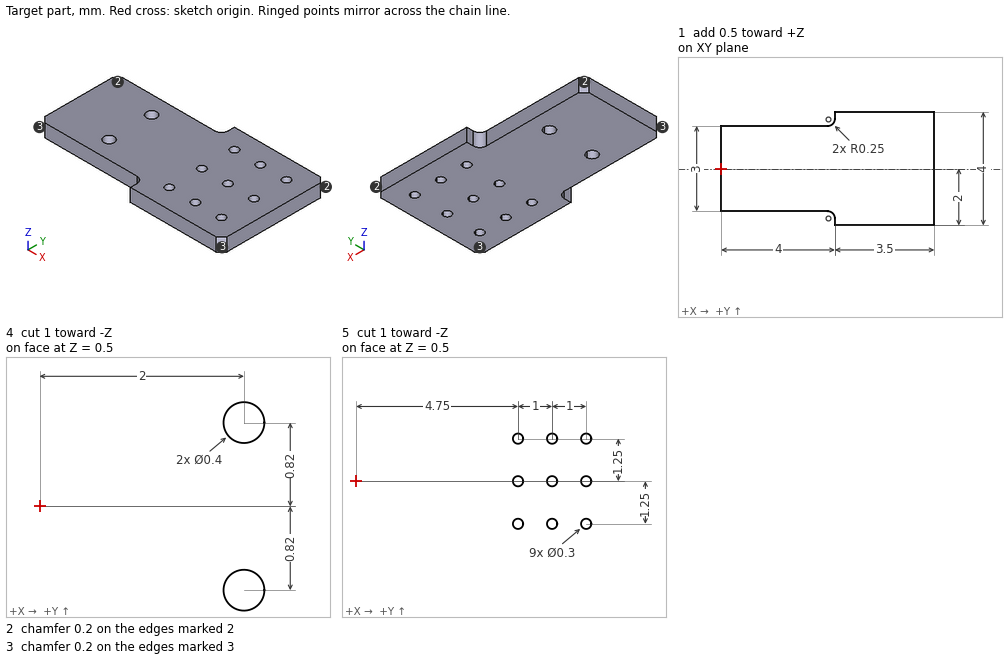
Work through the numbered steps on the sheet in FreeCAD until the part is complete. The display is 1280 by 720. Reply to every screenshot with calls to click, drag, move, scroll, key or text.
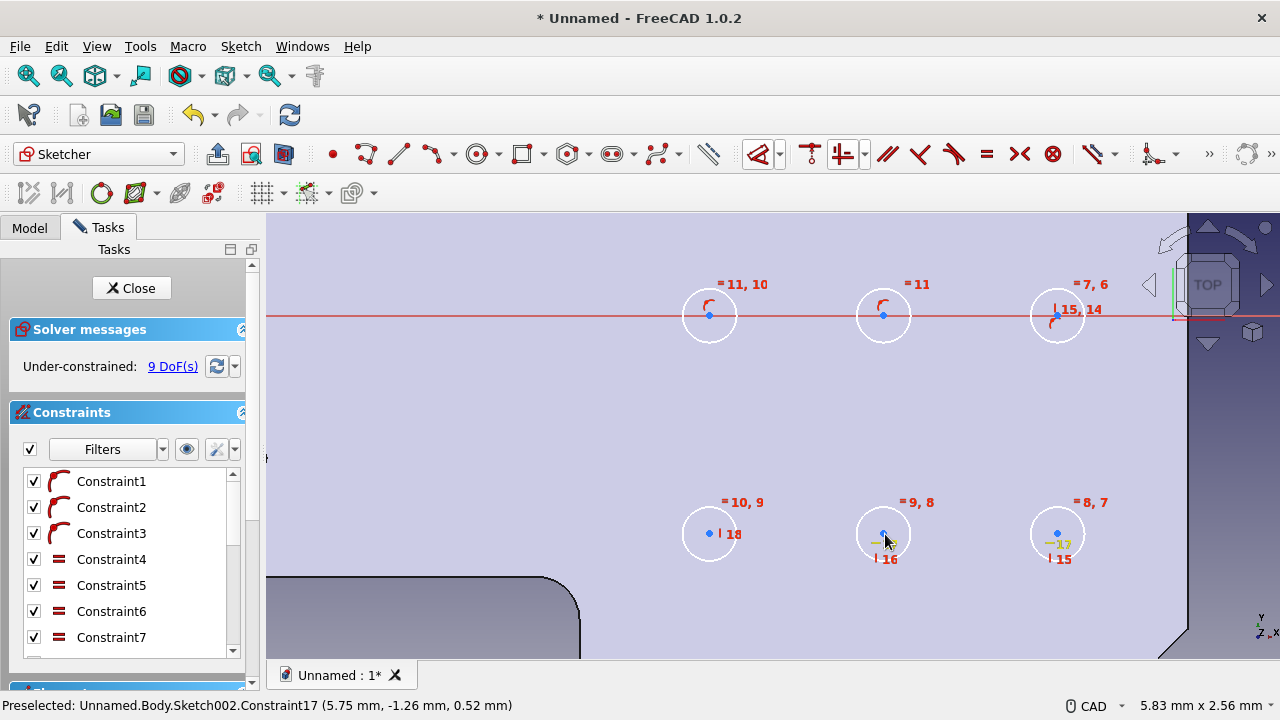
click(884, 534)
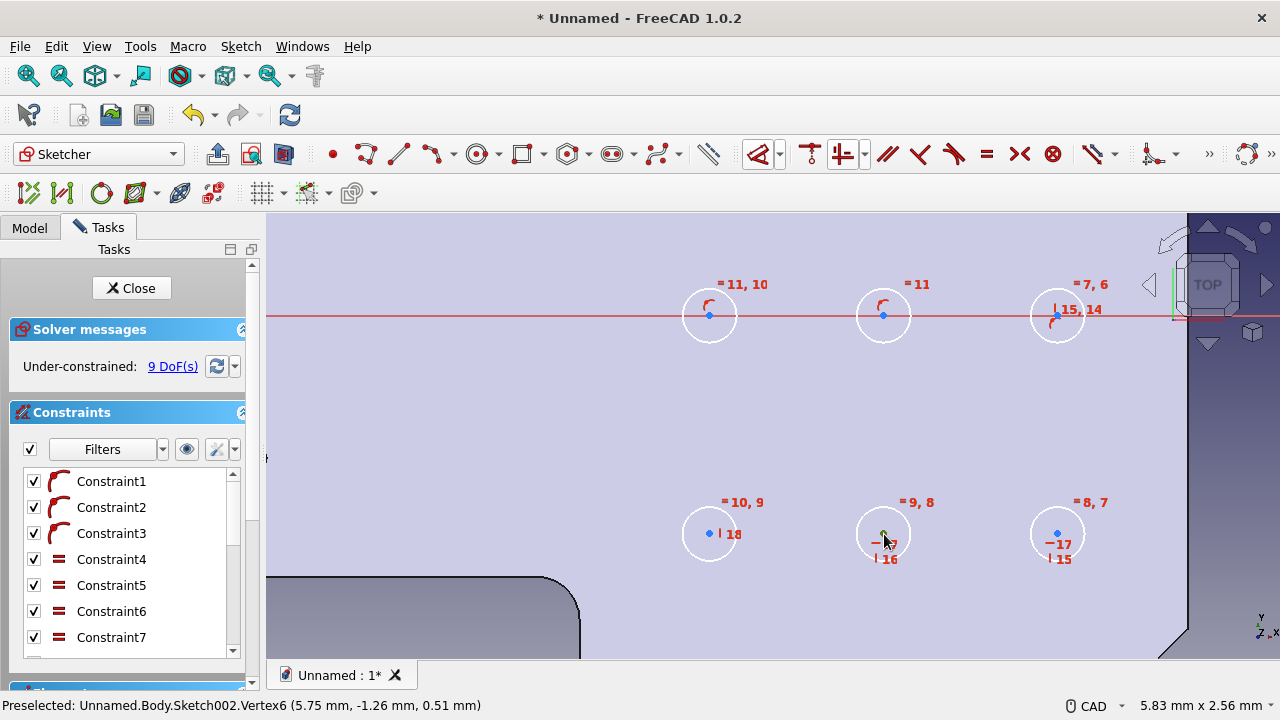
click(710, 534)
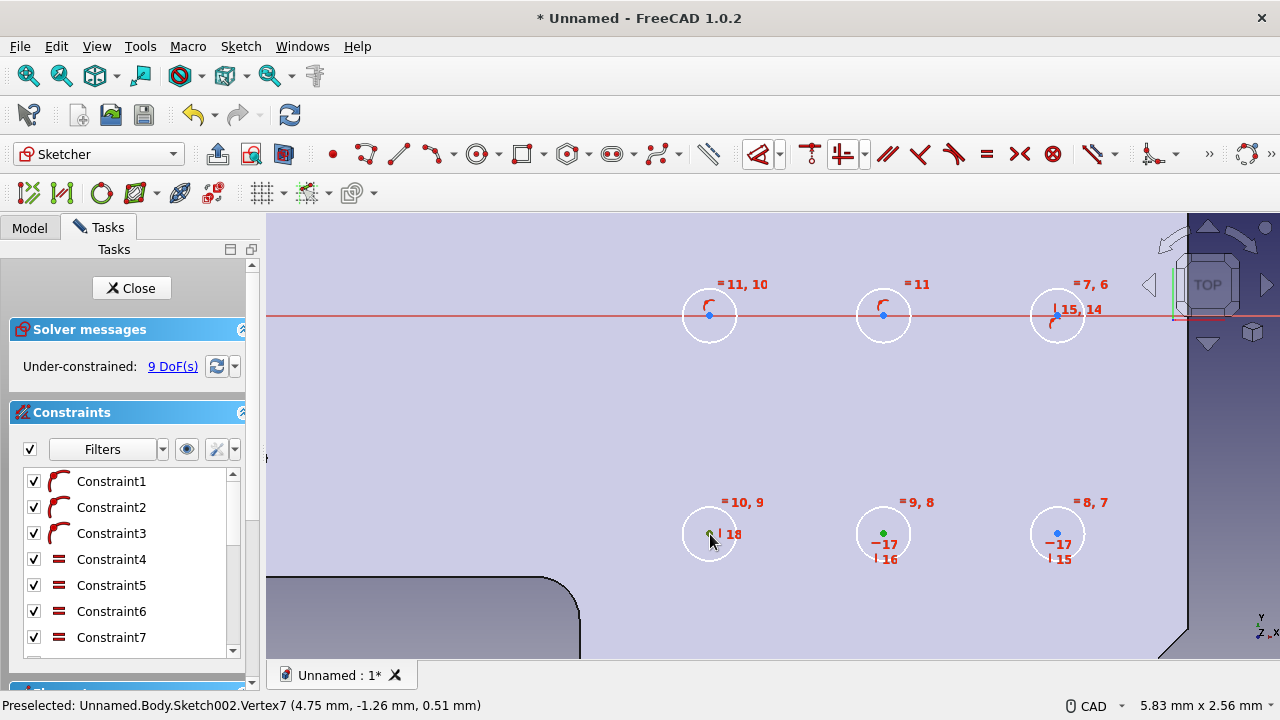
key(h)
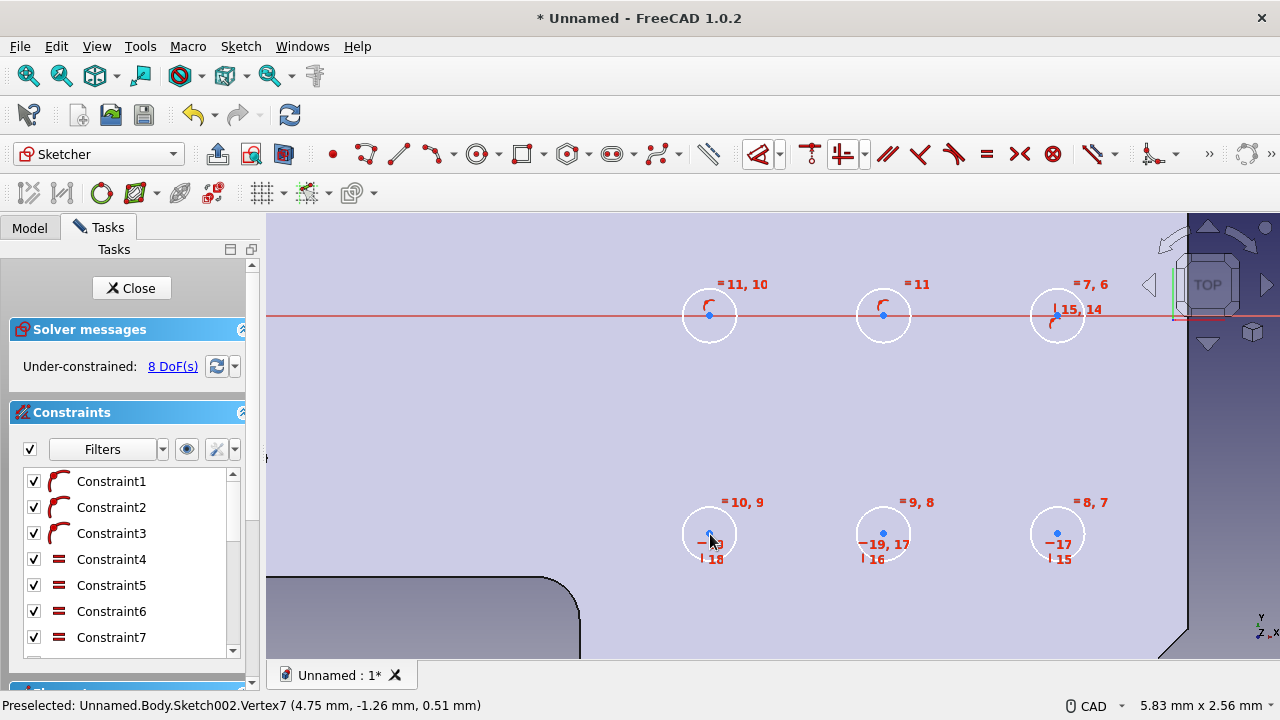
scroll(884, 534, down, 4)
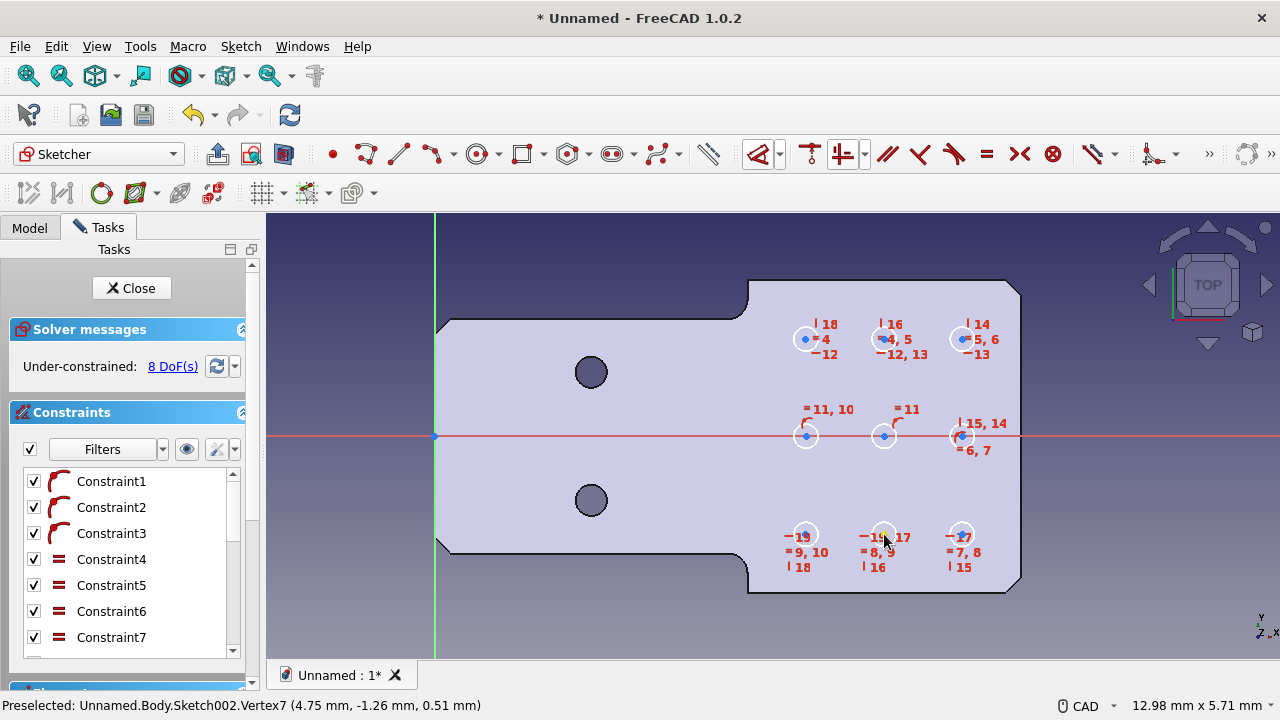
click(806, 339)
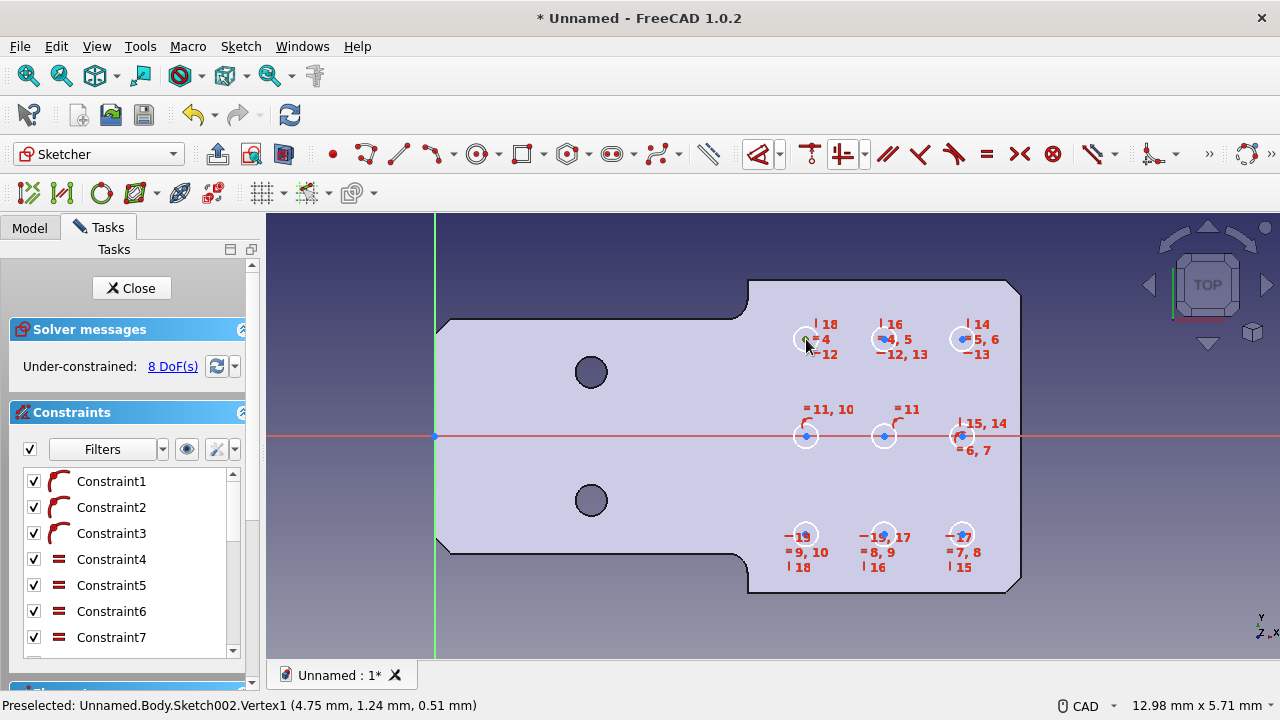
click(806, 436)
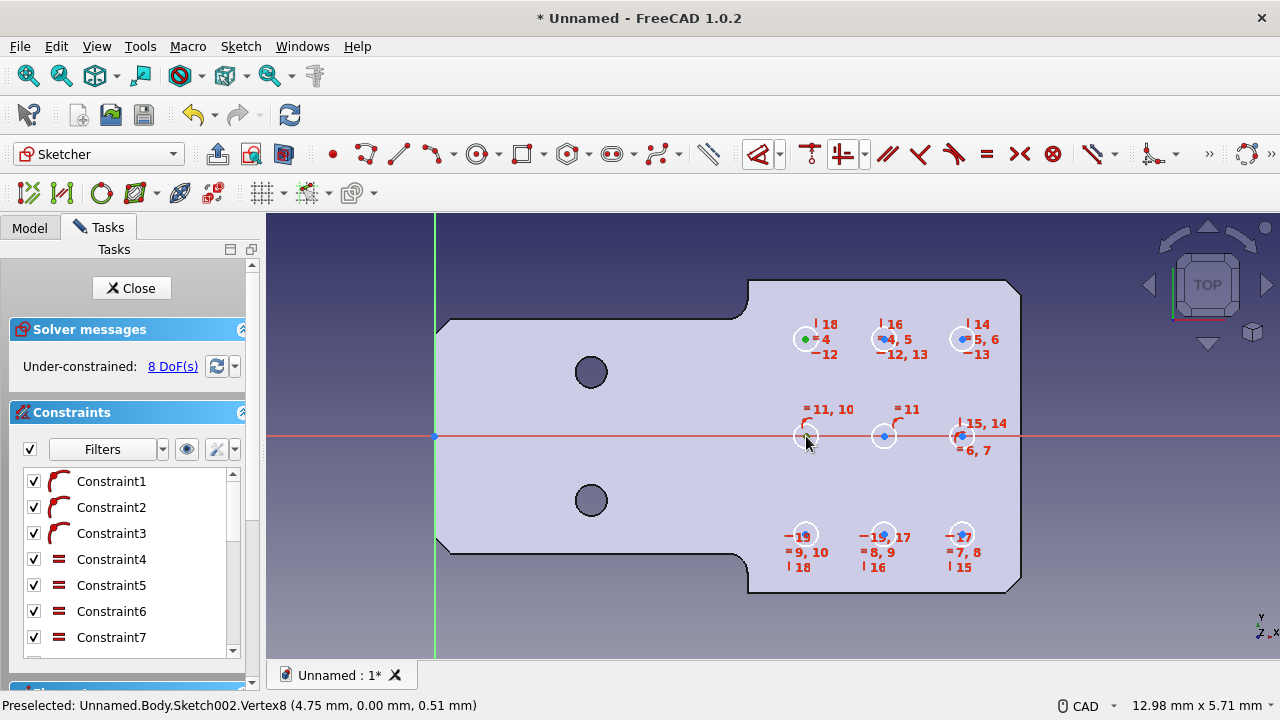
key(v)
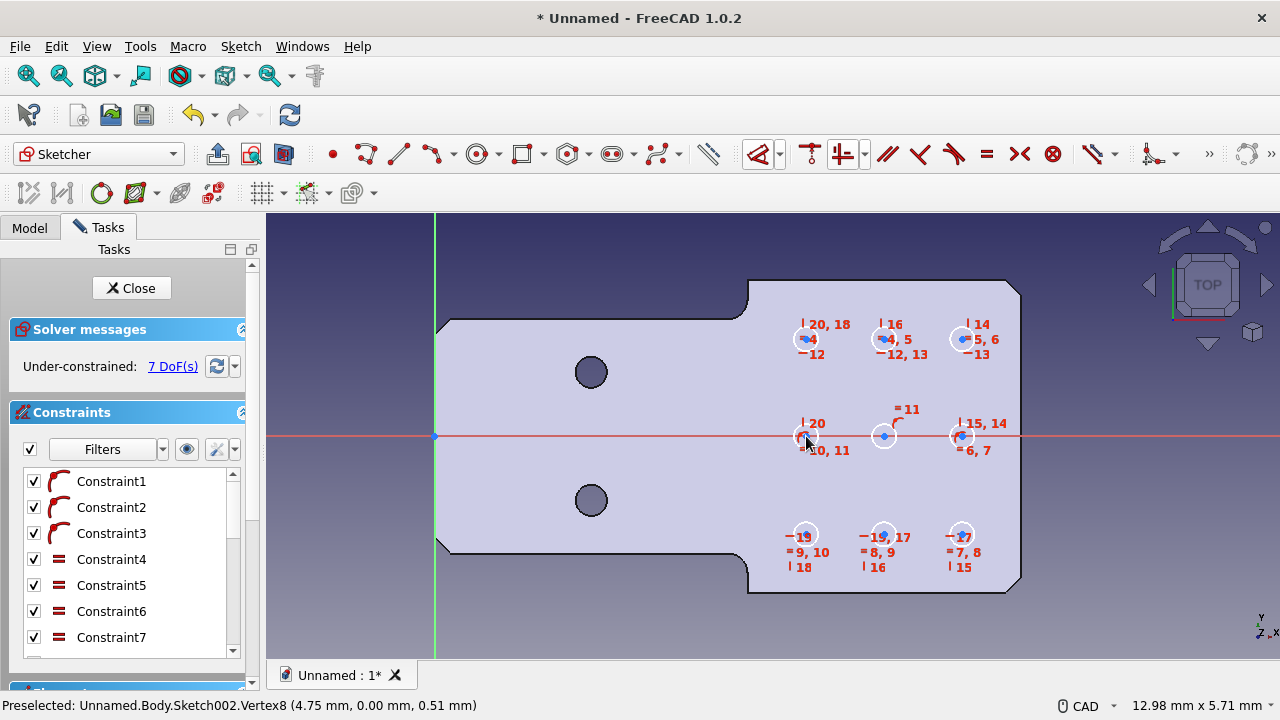
click(884, 339)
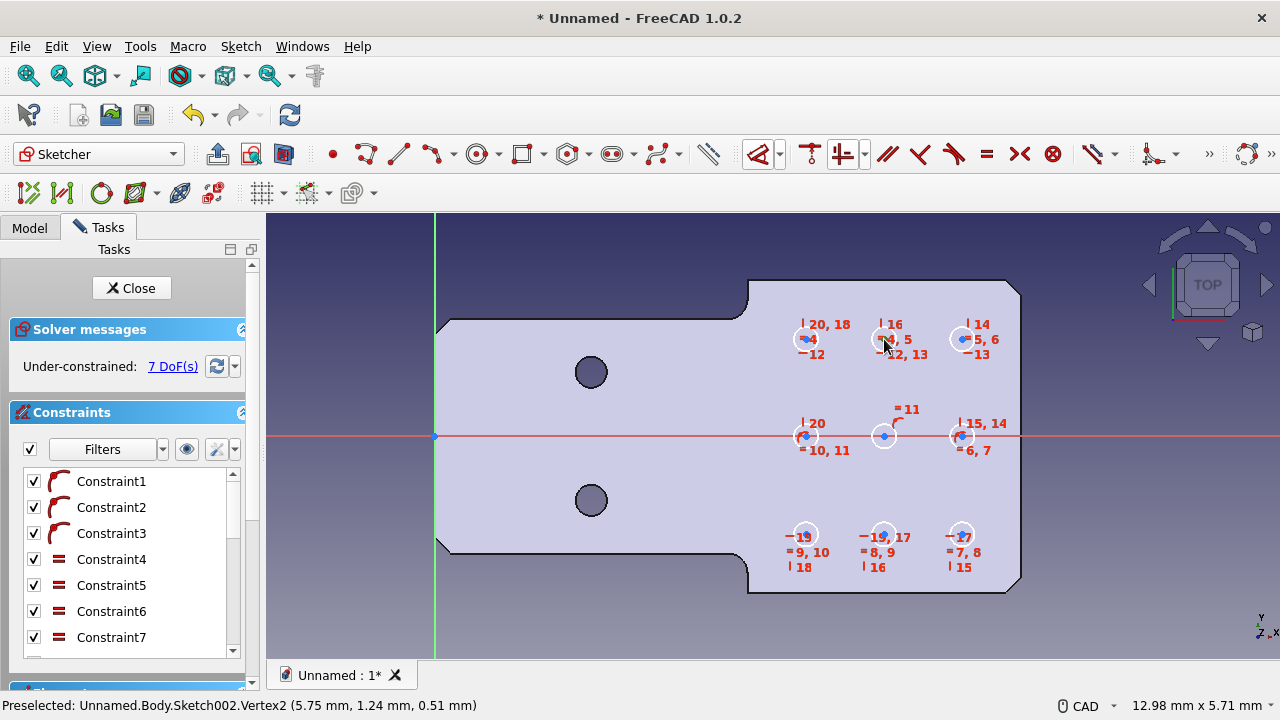
click(884, 436)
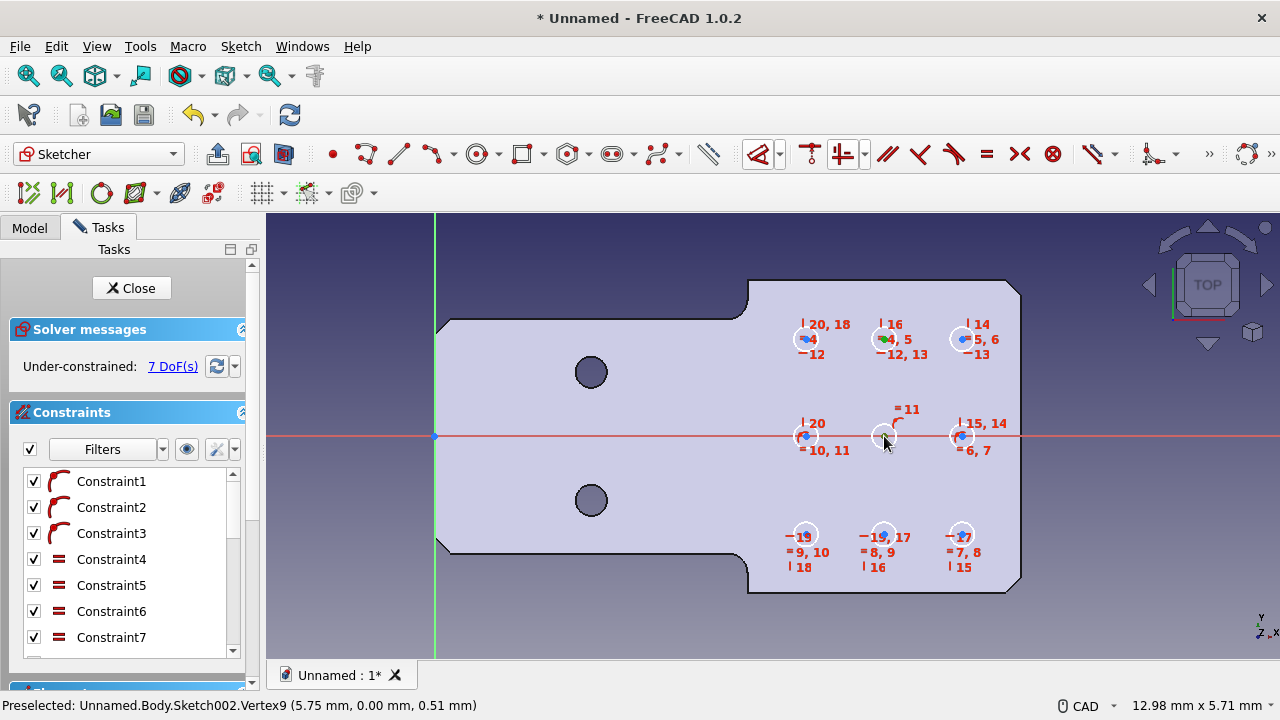
click(864, 154)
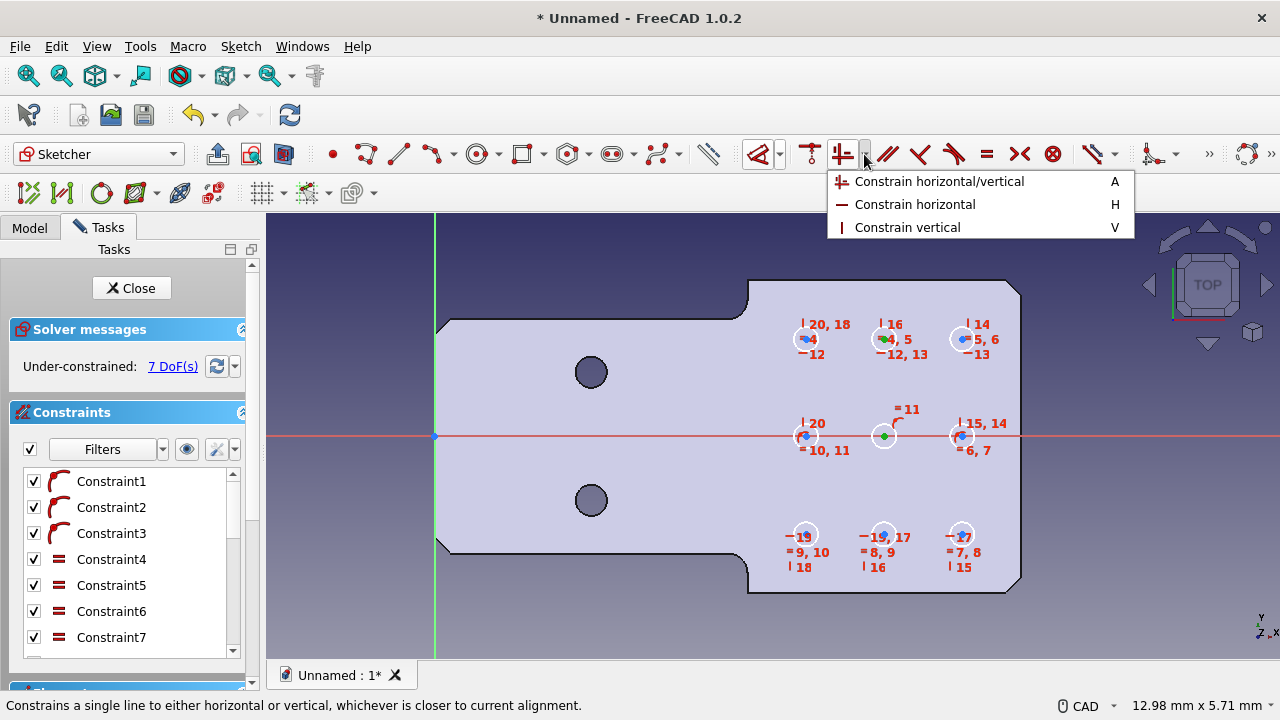
click(981, 228)